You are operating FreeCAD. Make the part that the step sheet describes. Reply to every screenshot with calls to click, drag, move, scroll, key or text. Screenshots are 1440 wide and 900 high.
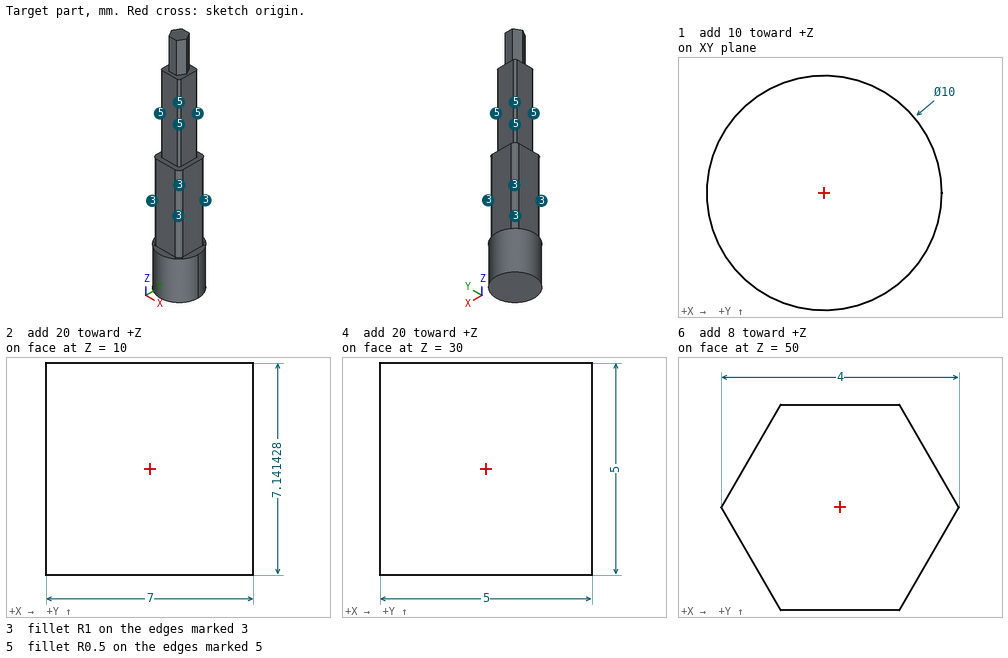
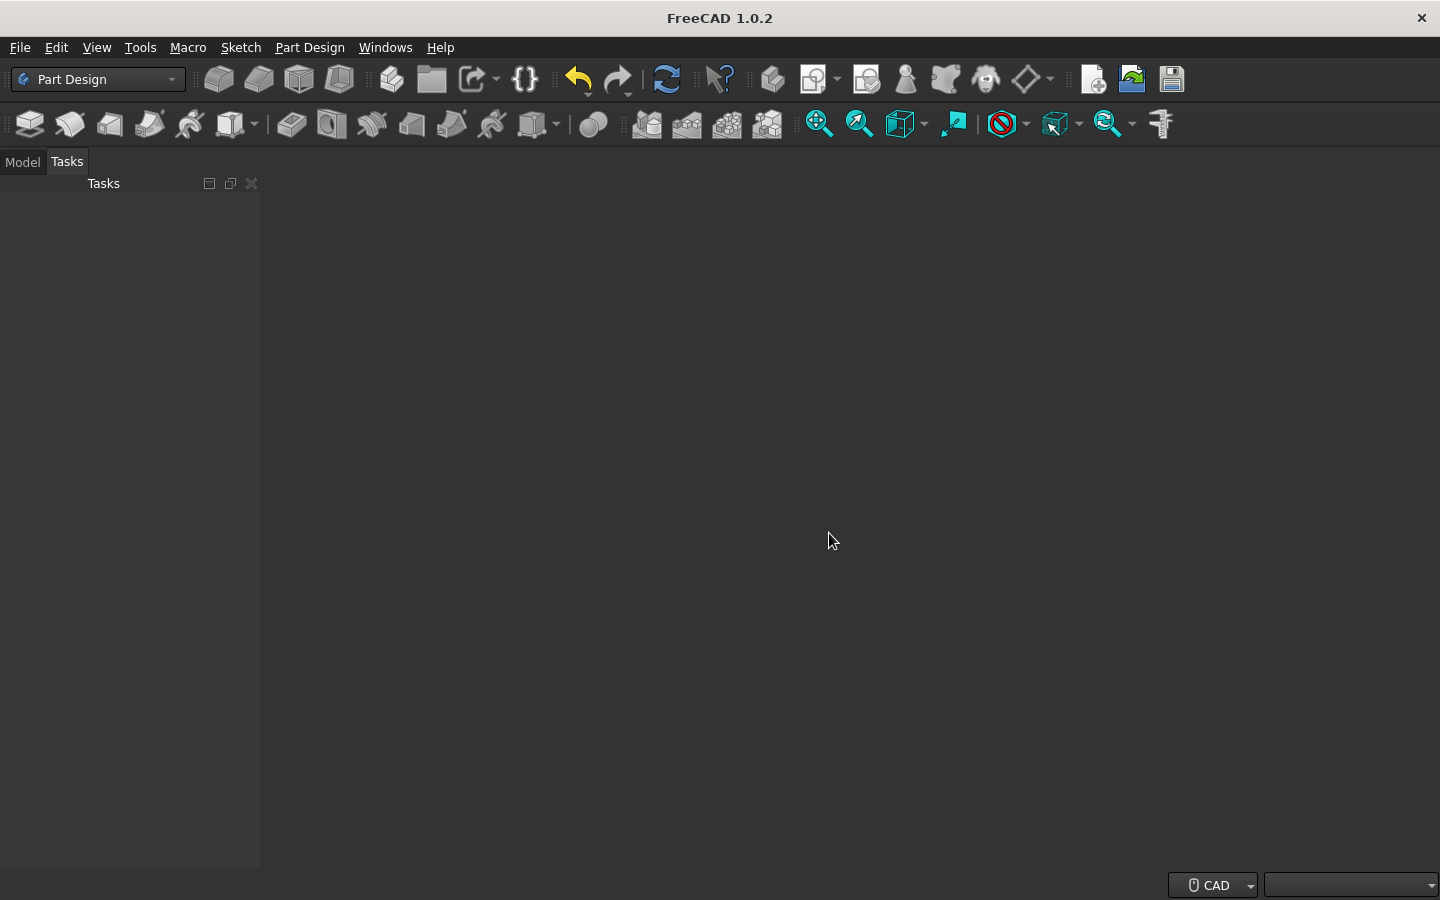
click(1092, 80)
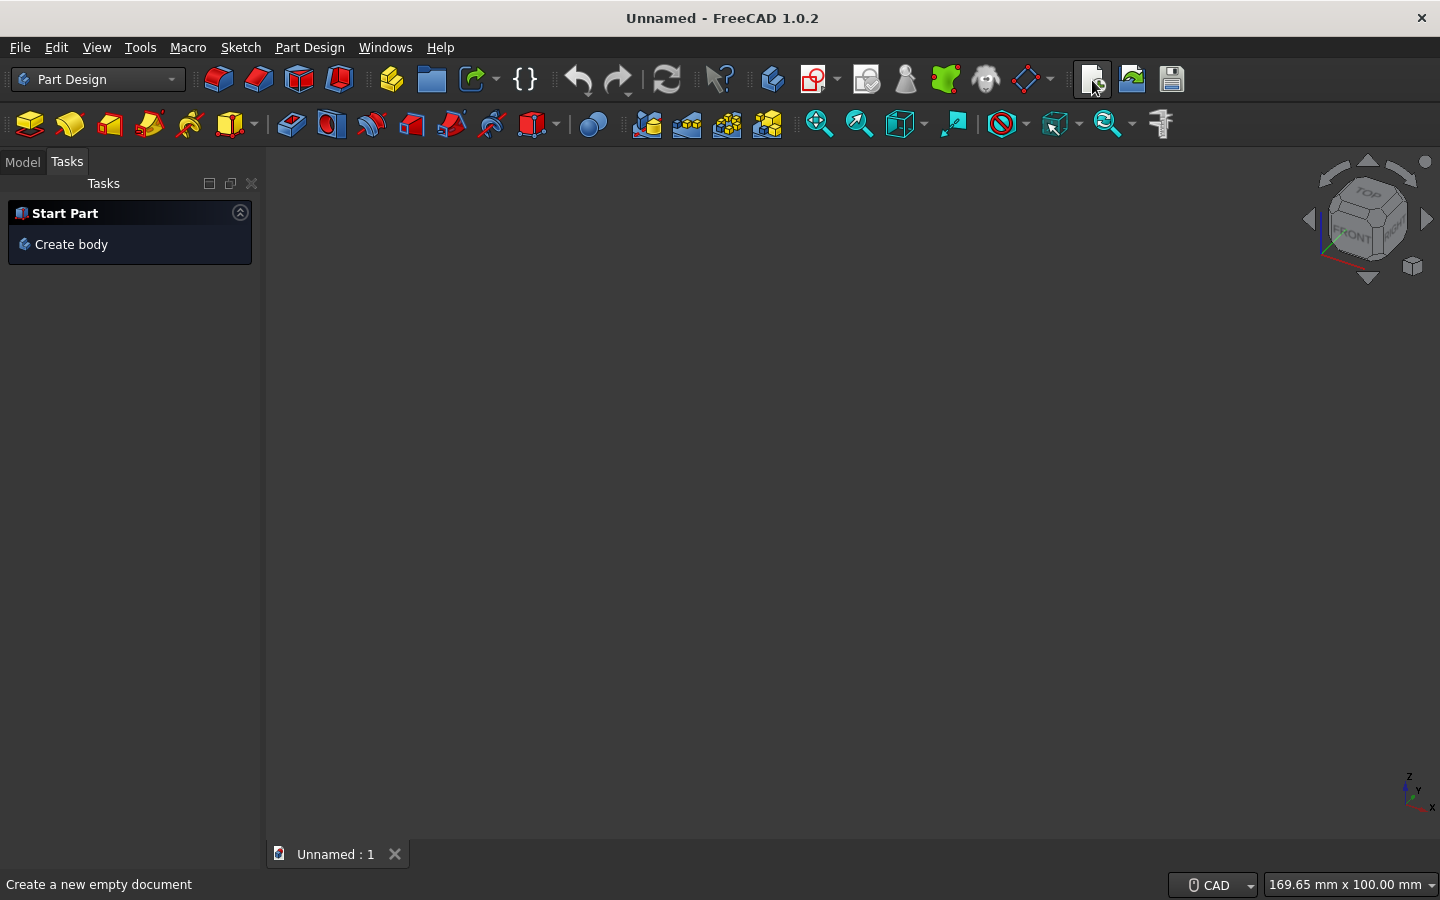
click(814, 80)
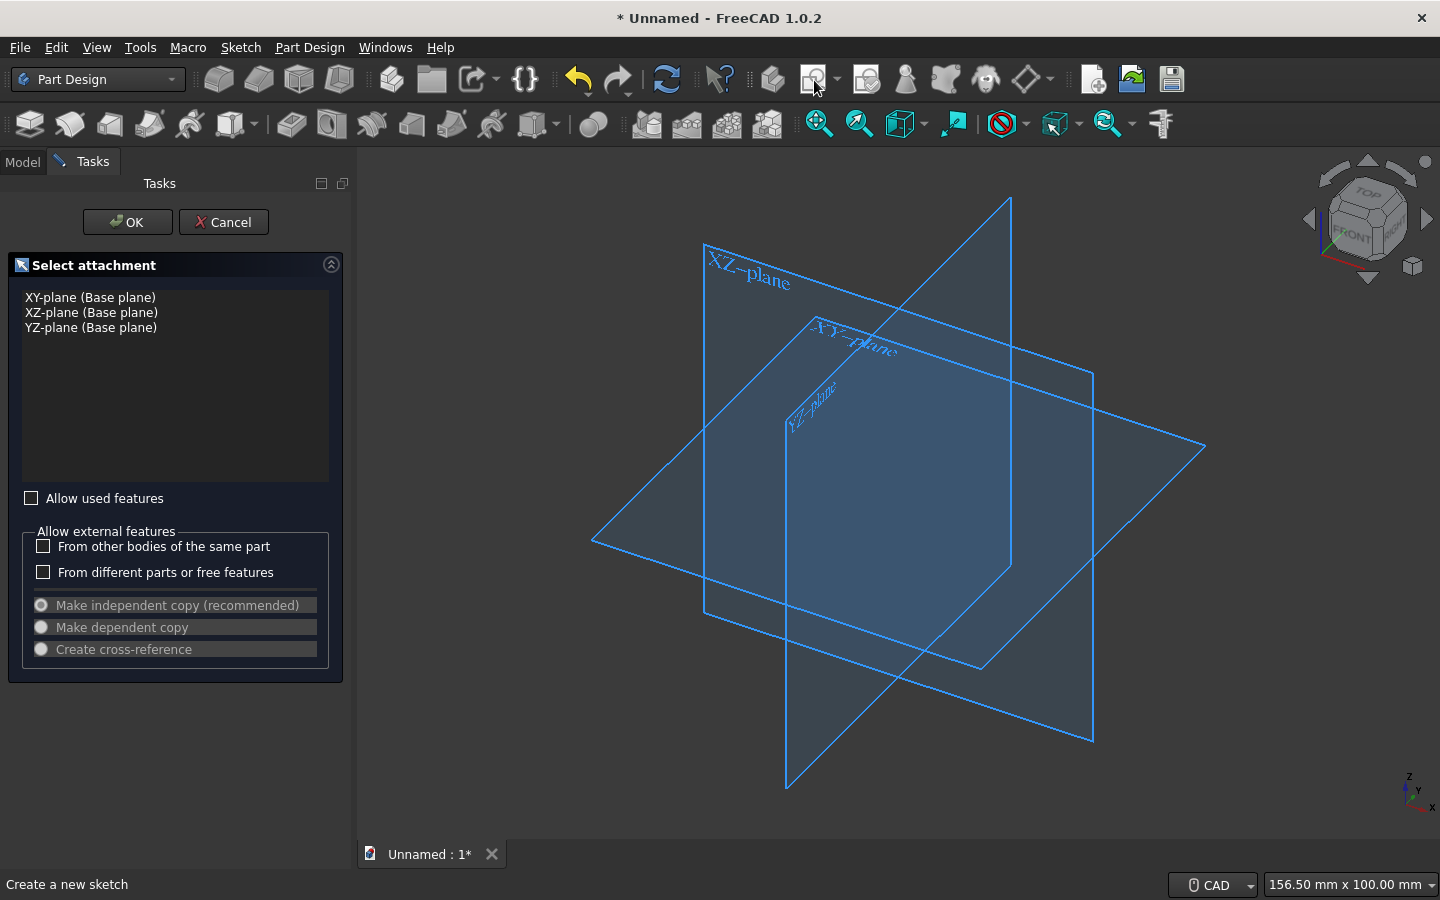
click(82, 298)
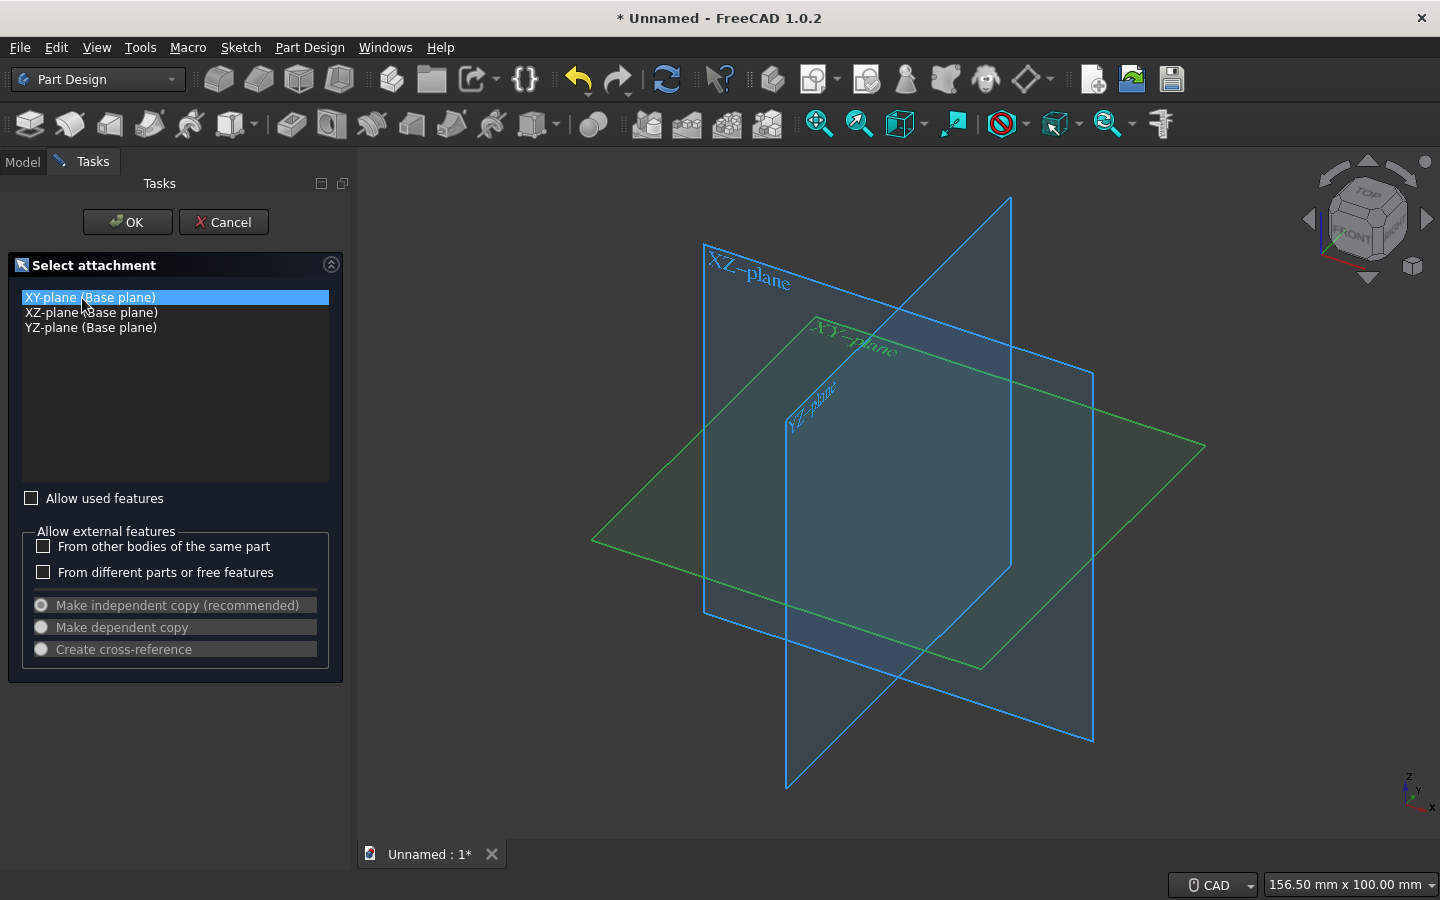
click(128, 222)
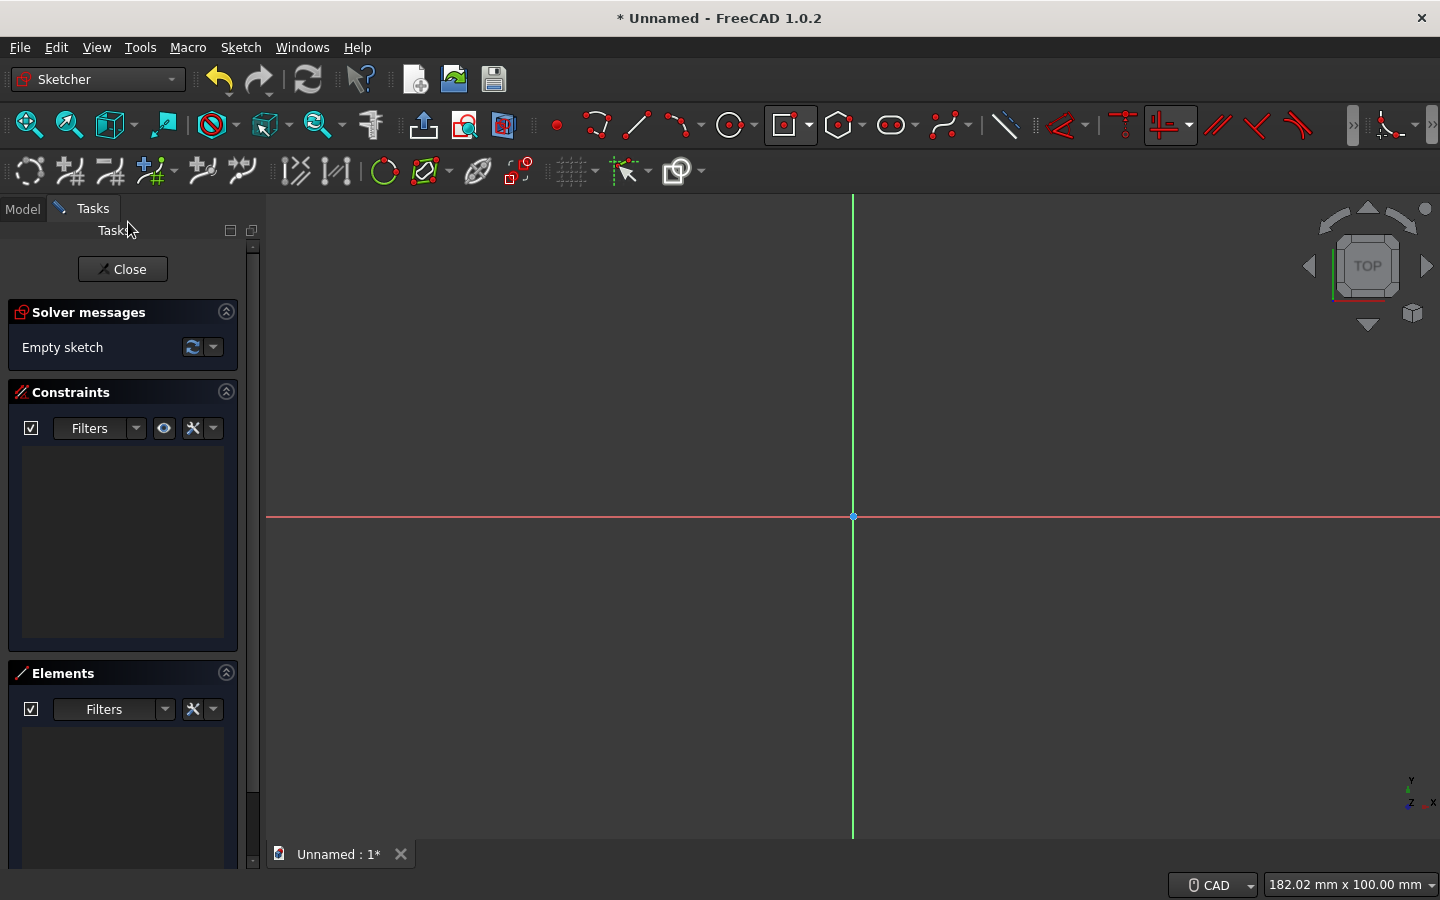
scroll(867, 516, up, 9)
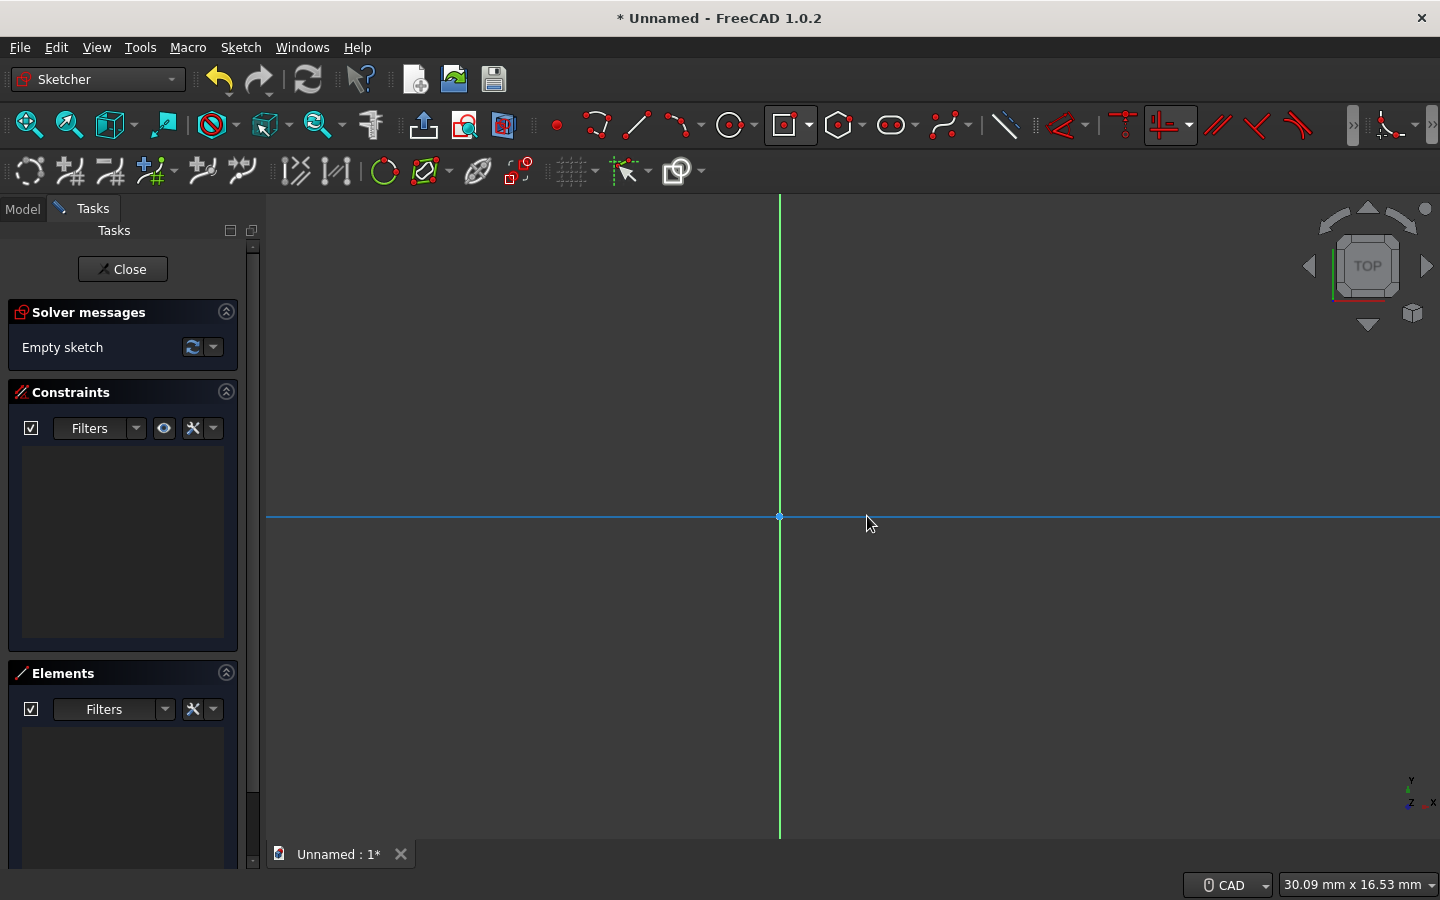
click(730, 126)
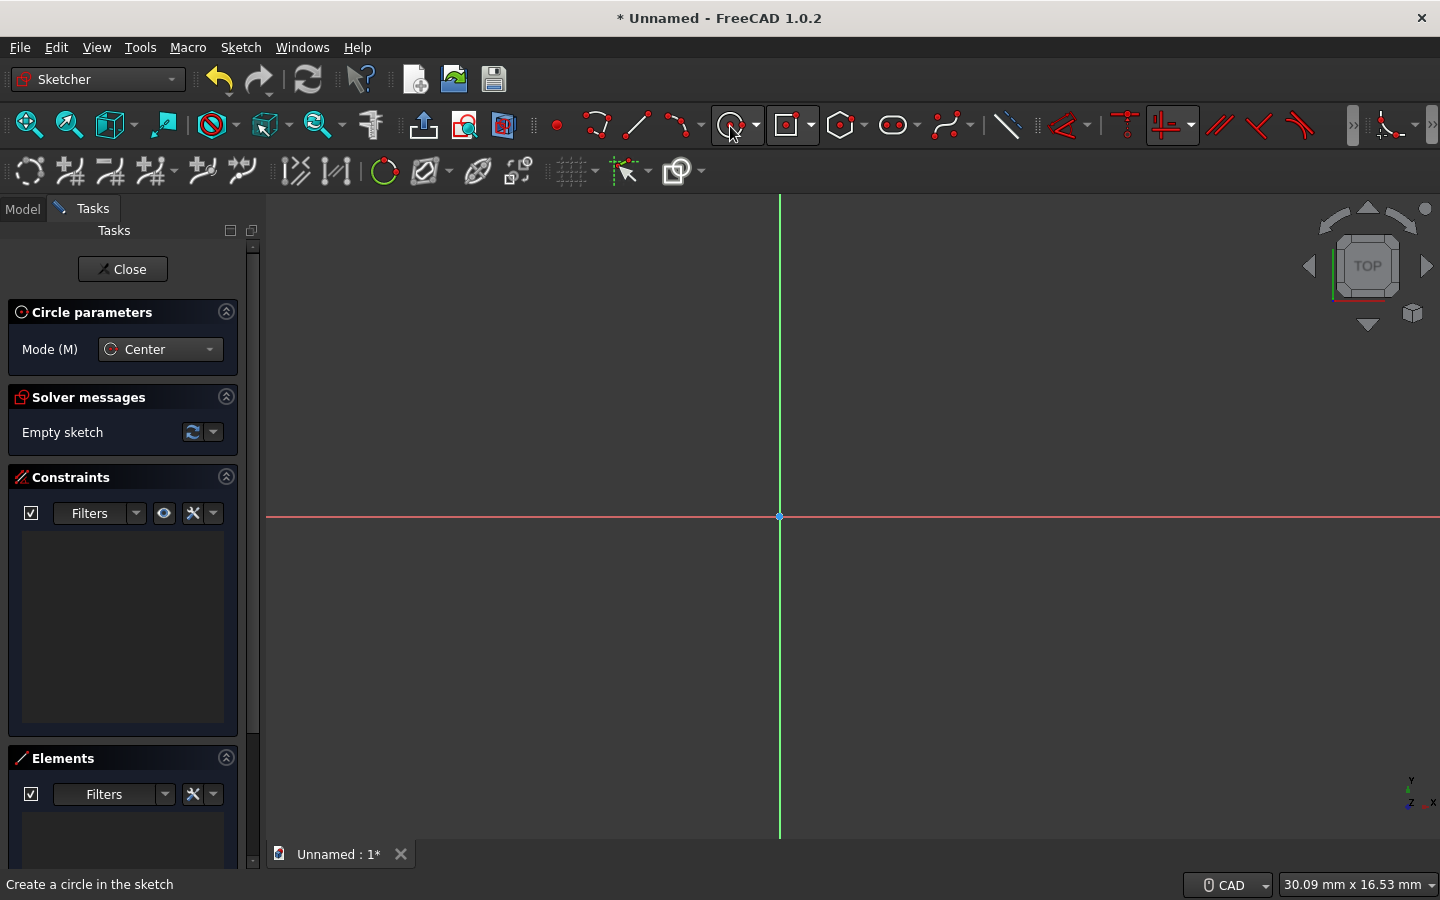
click(780, 516)
click(918, 379)
key(Escape)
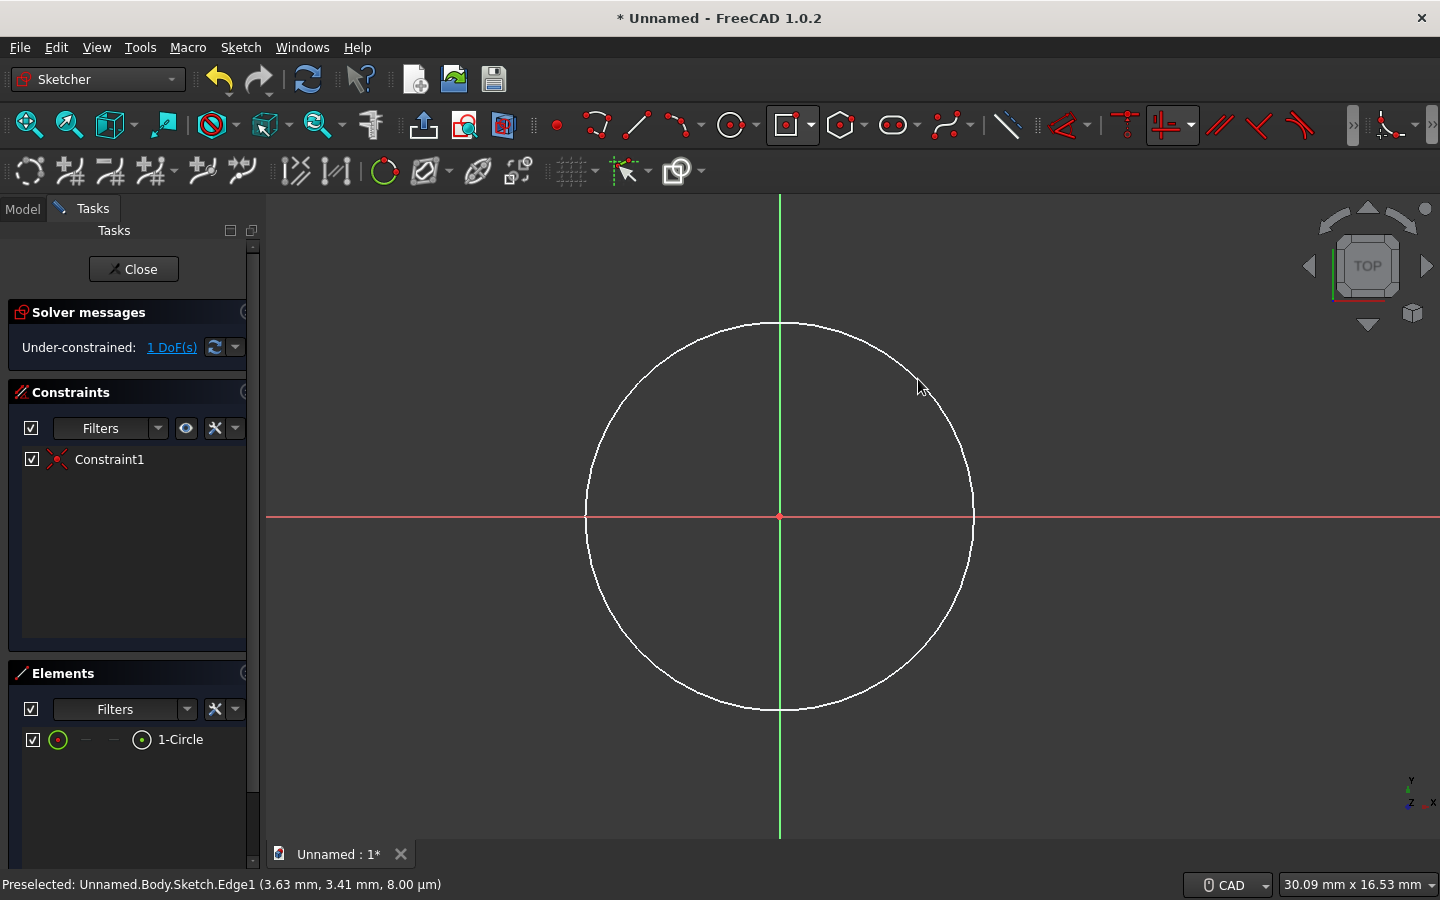
click(1062, 126)